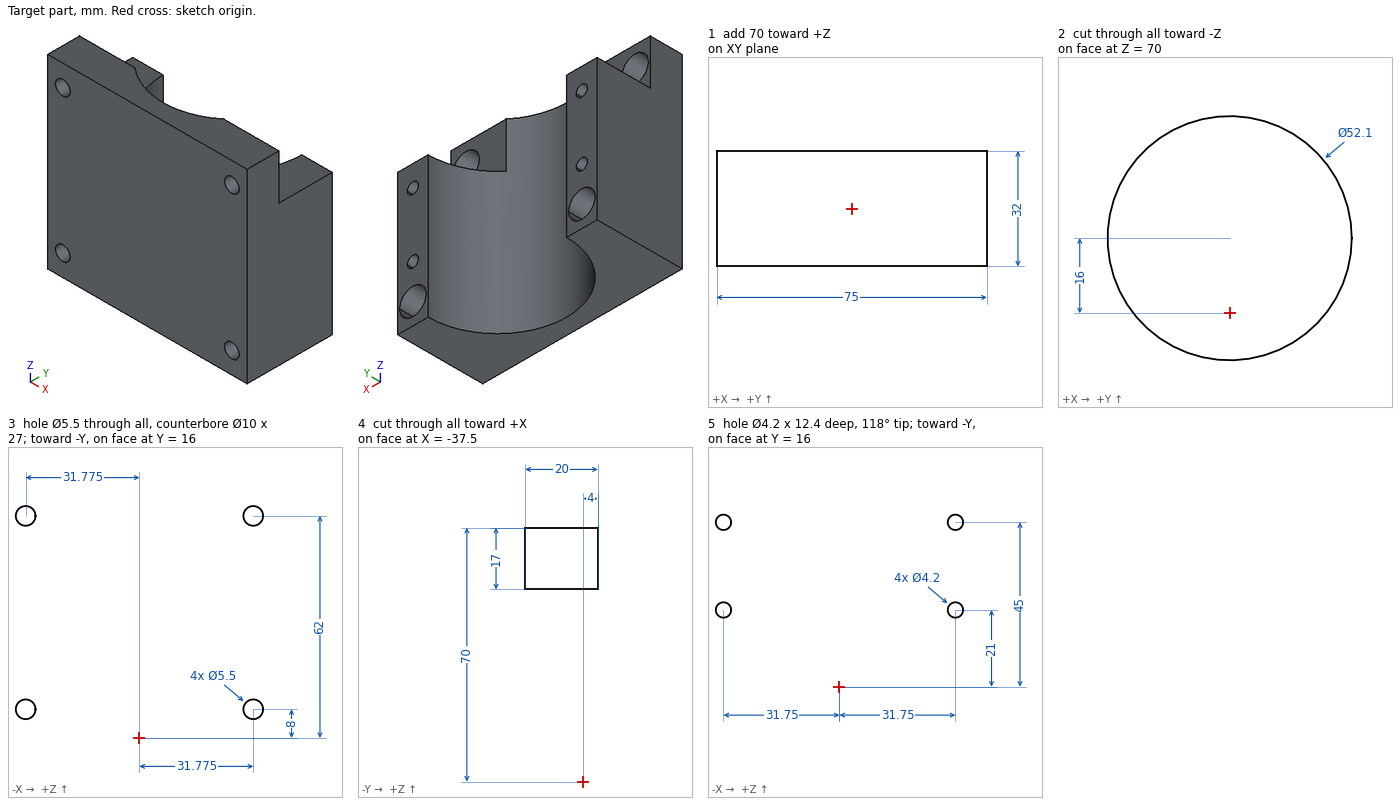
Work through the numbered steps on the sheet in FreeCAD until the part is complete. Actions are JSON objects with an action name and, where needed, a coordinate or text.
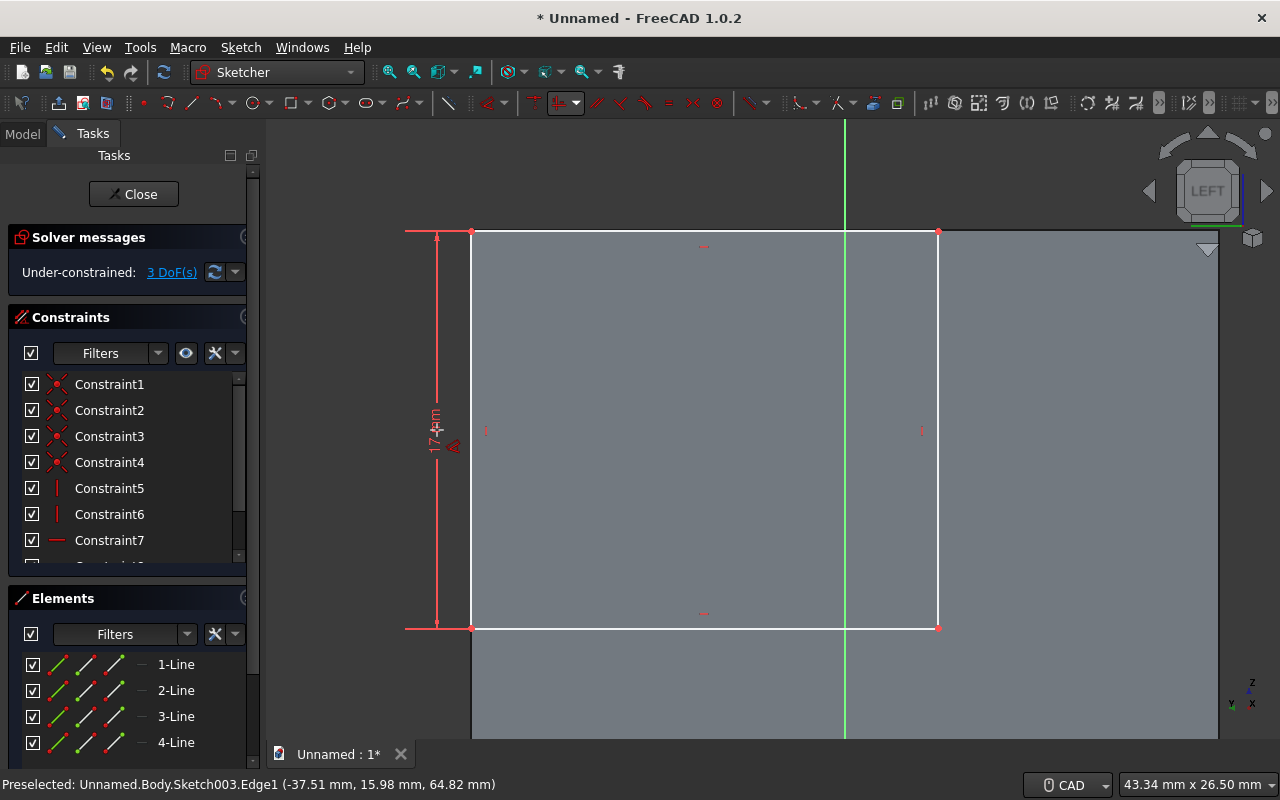
{"action": "left_click", "coordinate": [611, 629]}
{"action": "left_click", "coordinate": [705, 663]}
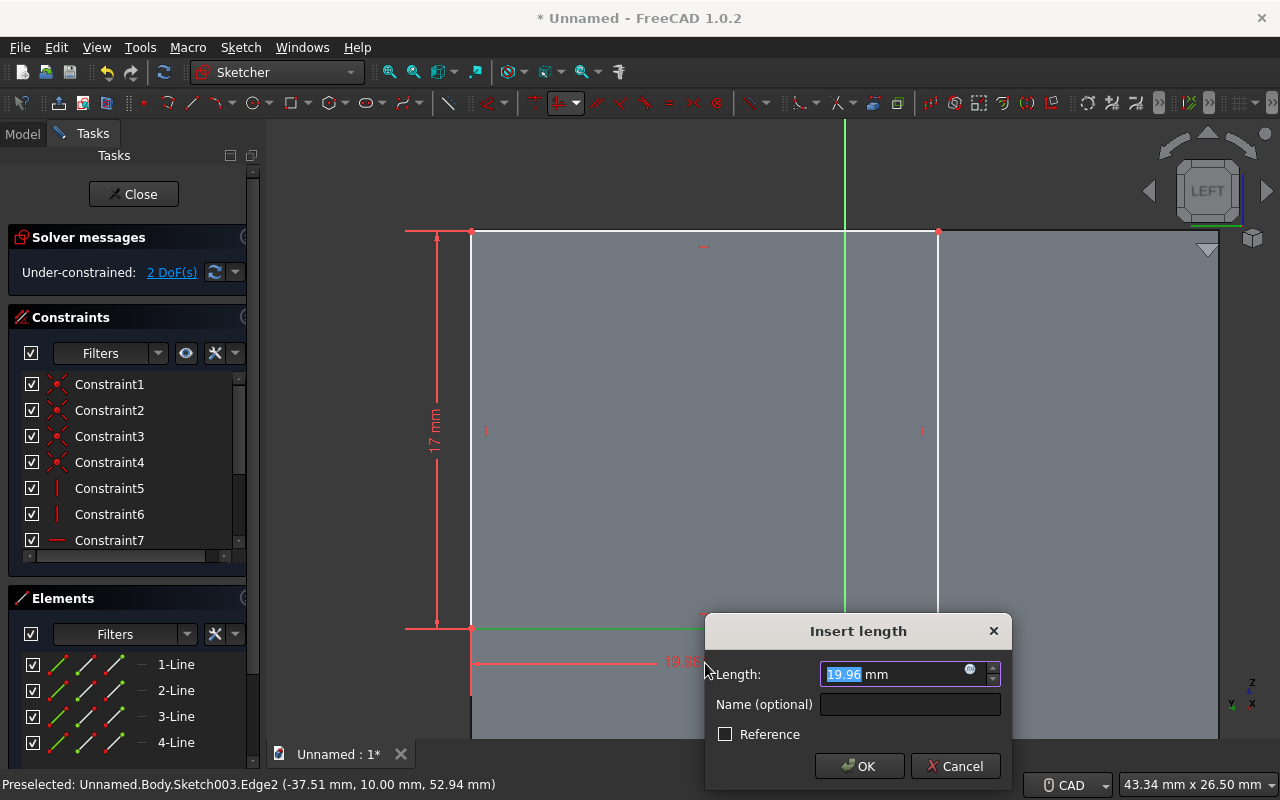
{"action": "type", "text": "20"}
{"action": "key", "text": "Return"}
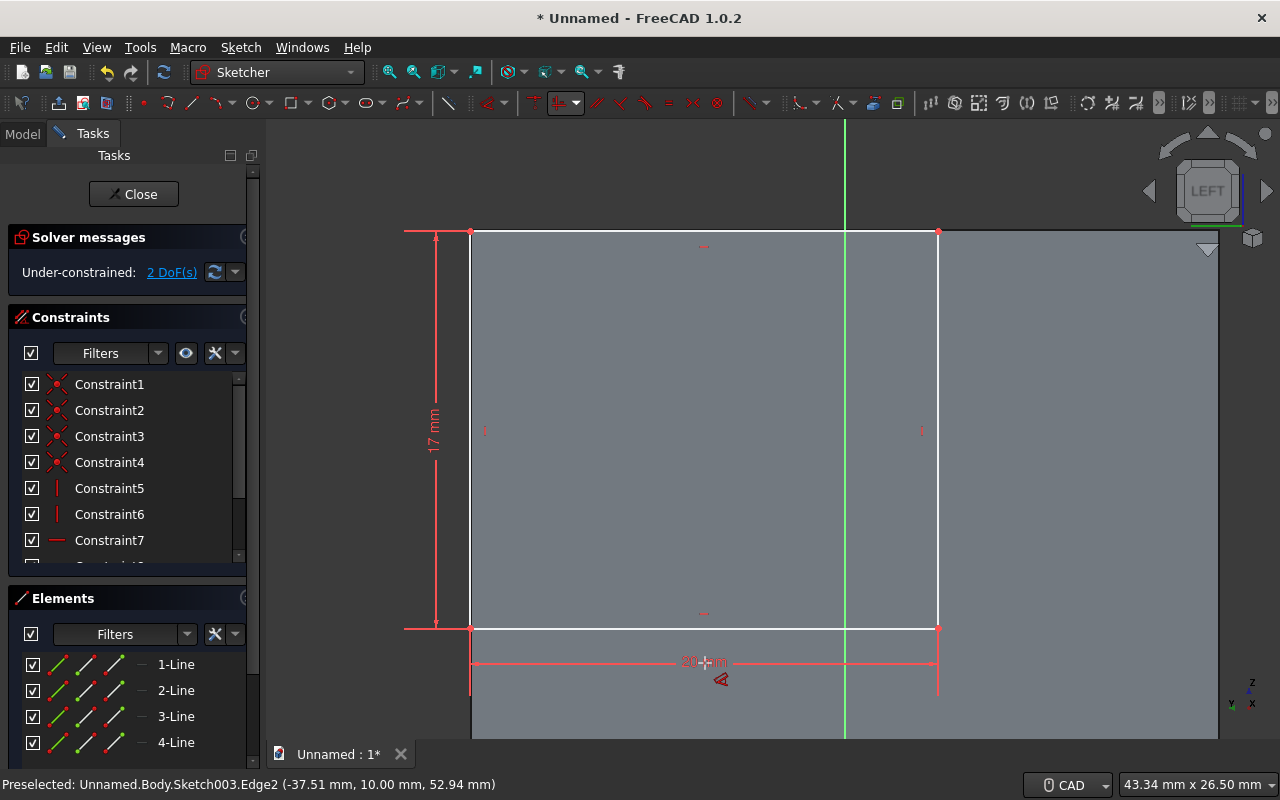
{"action": "left_click", "coordinate": [938, 629]}
{"action": "left_click", "coordinate": [891, 595]}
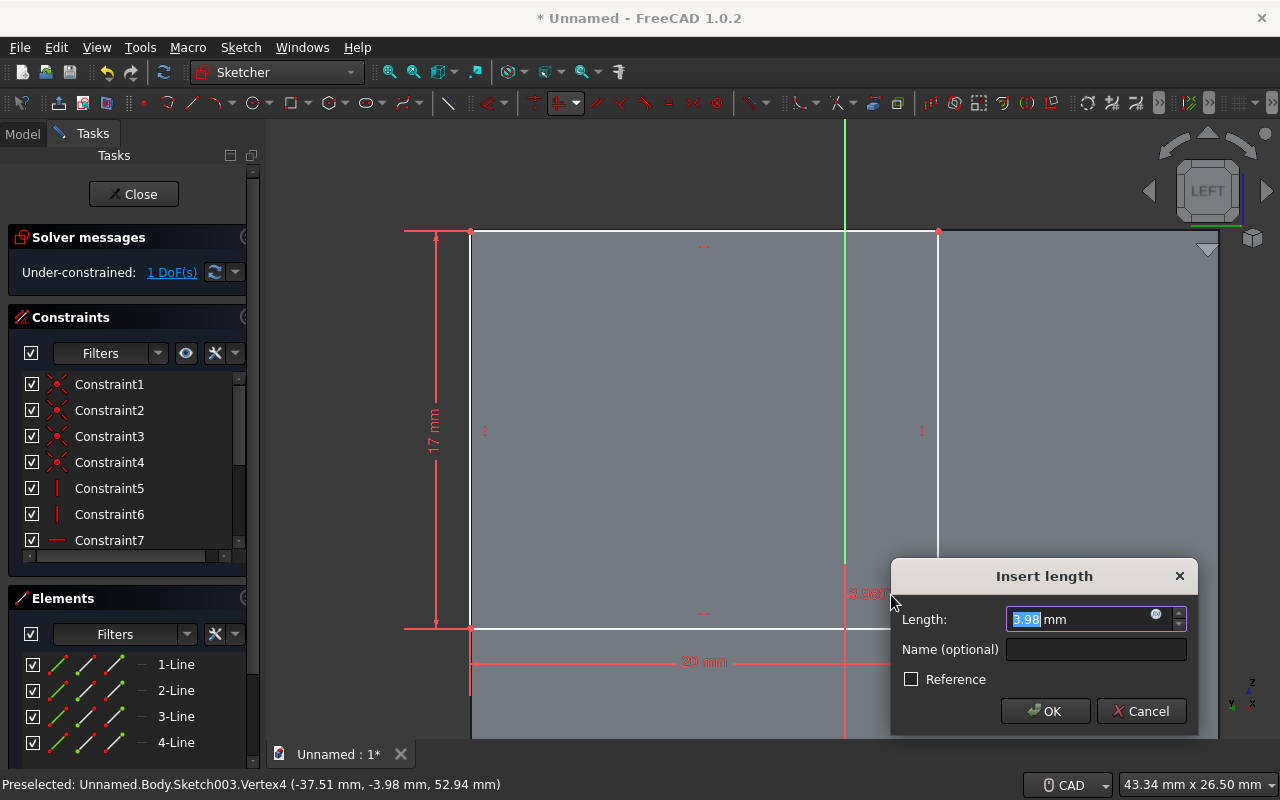
{"action": "type", "text": "4"}
{"action": "key", "text": "Return"}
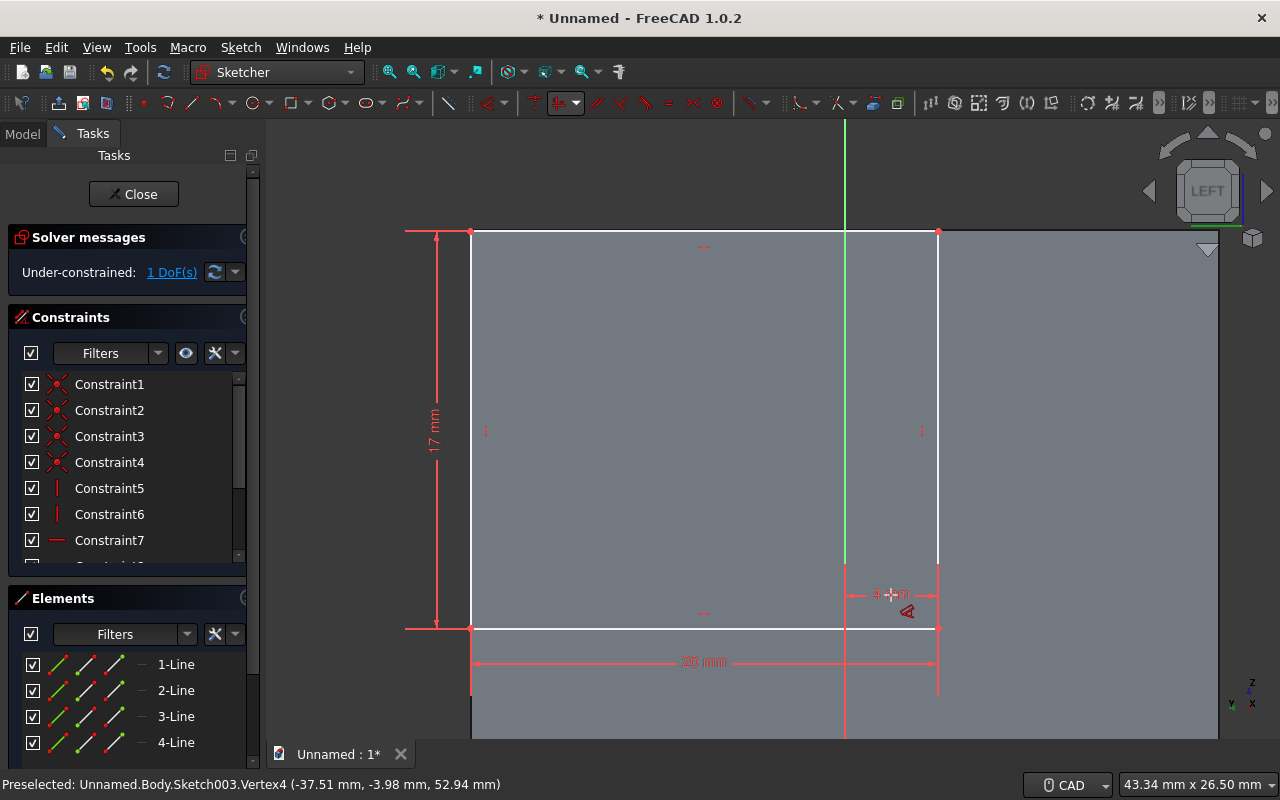
{"action": "left_click", "coordinate": [471, 231]}
{"action": "left_click", "coordinate": [437, 471]}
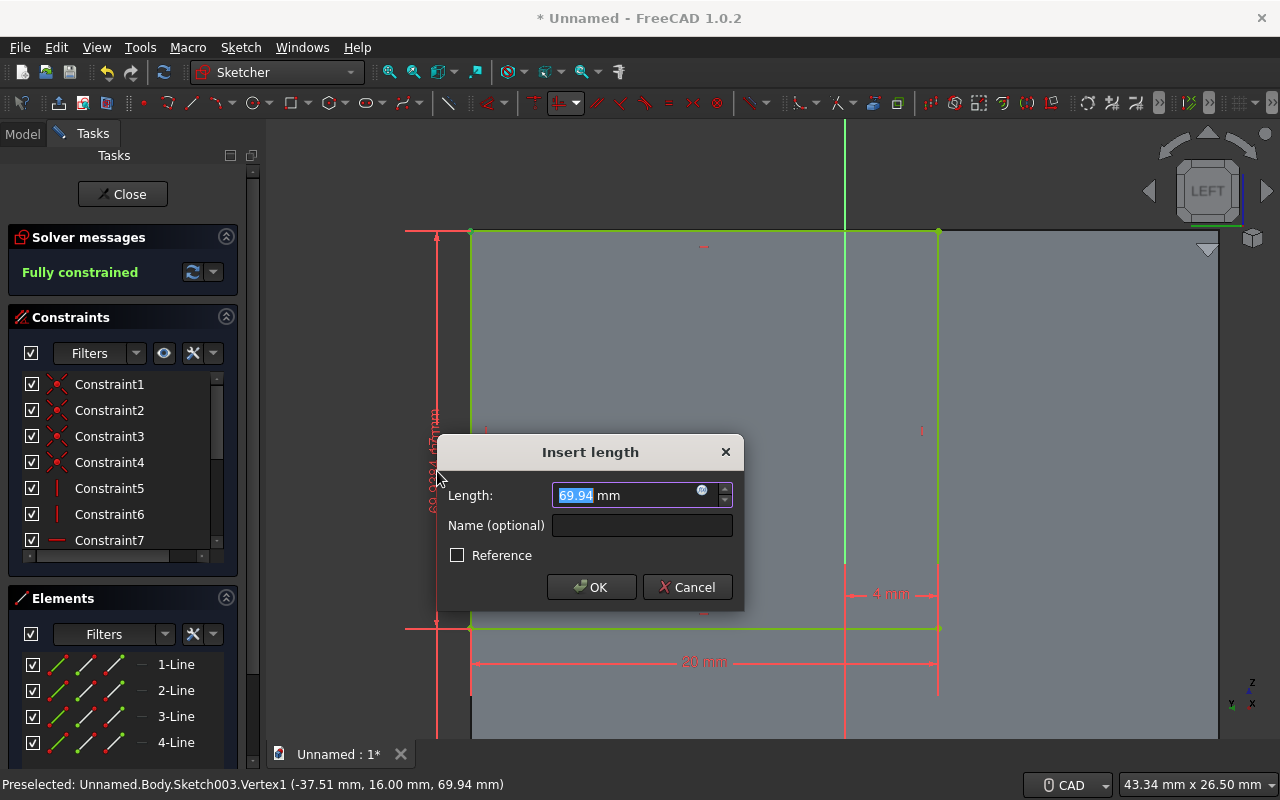
{"action": "type", "text": "70"}
{"action": "key", "text": "Return"}
{"action": "key", "text": "Escape"}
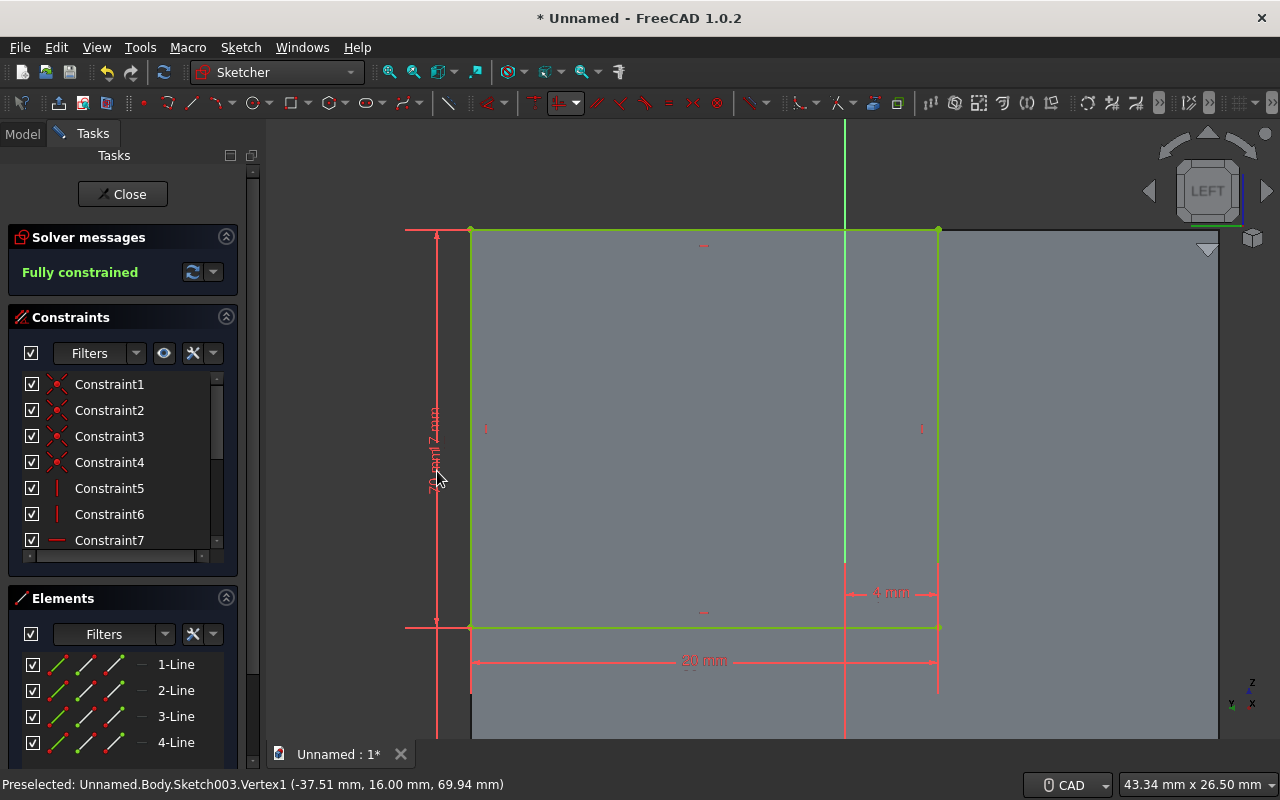
{"action": "left_click", "coordinate": [123, 194]}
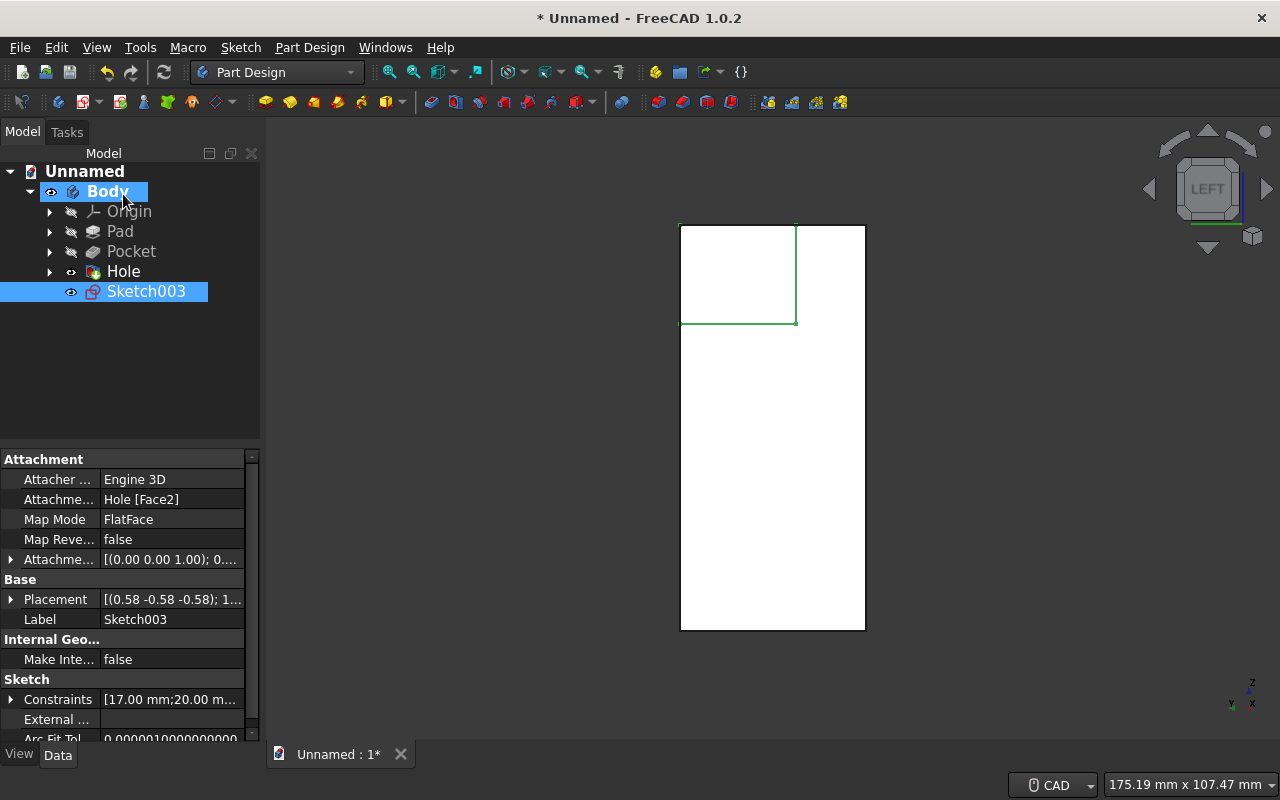
{"action": "left_click", "coordinate": [432, 102]}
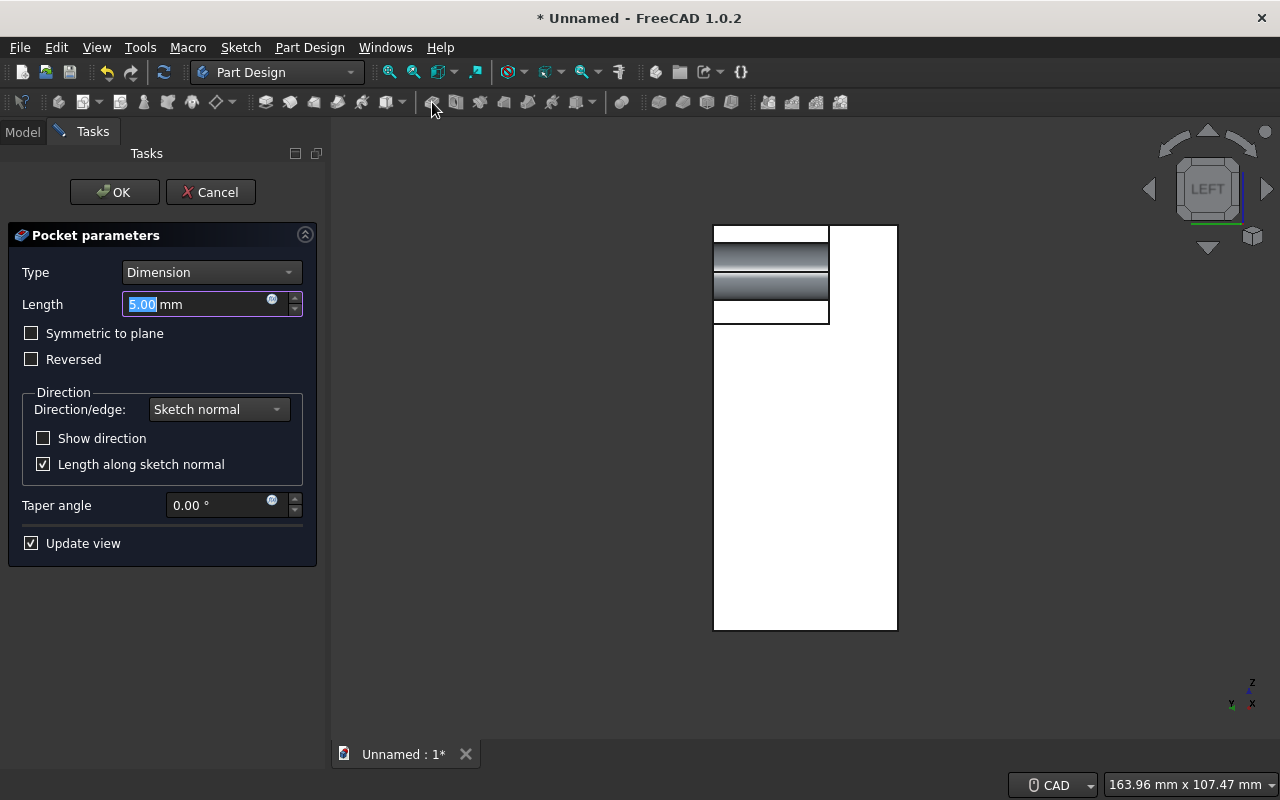
{"action": "left_click", "coordinate": [212, 272]}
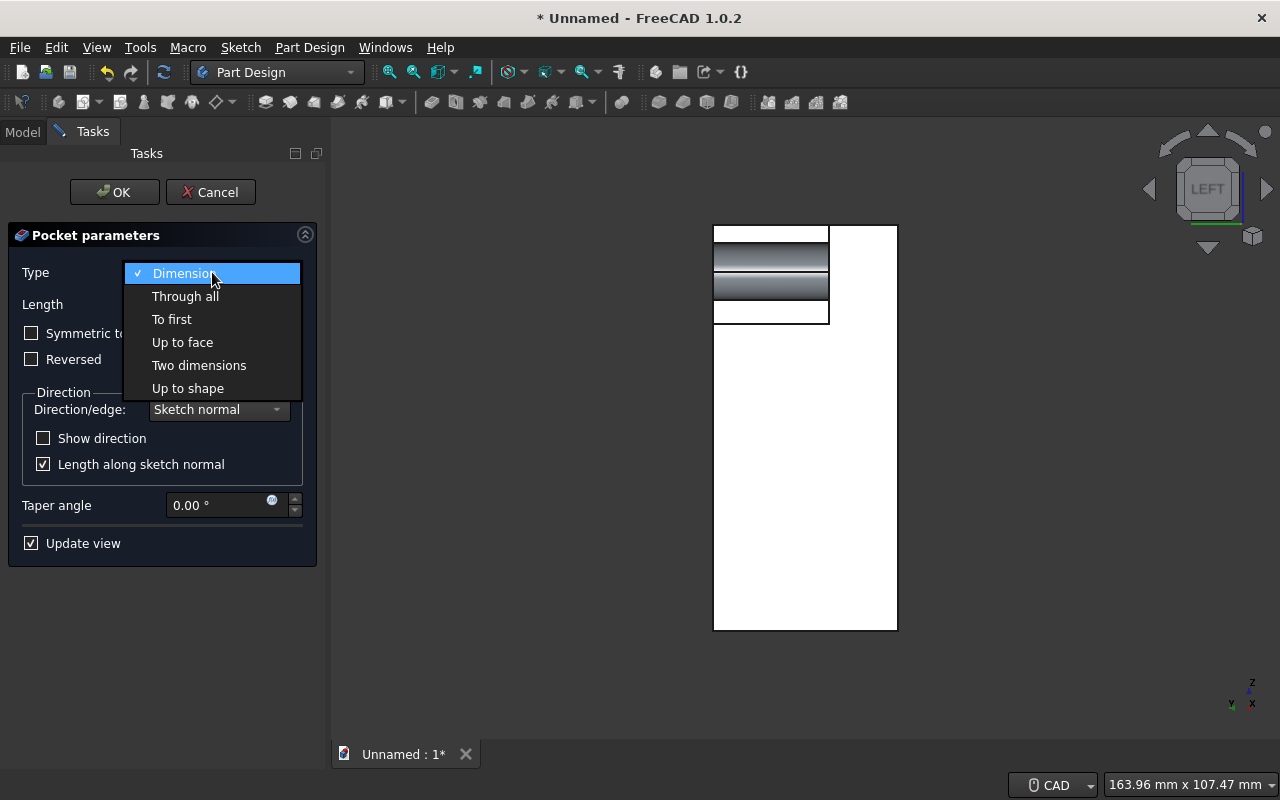
{"action": "left_click", "coordinate": [212, 296]}